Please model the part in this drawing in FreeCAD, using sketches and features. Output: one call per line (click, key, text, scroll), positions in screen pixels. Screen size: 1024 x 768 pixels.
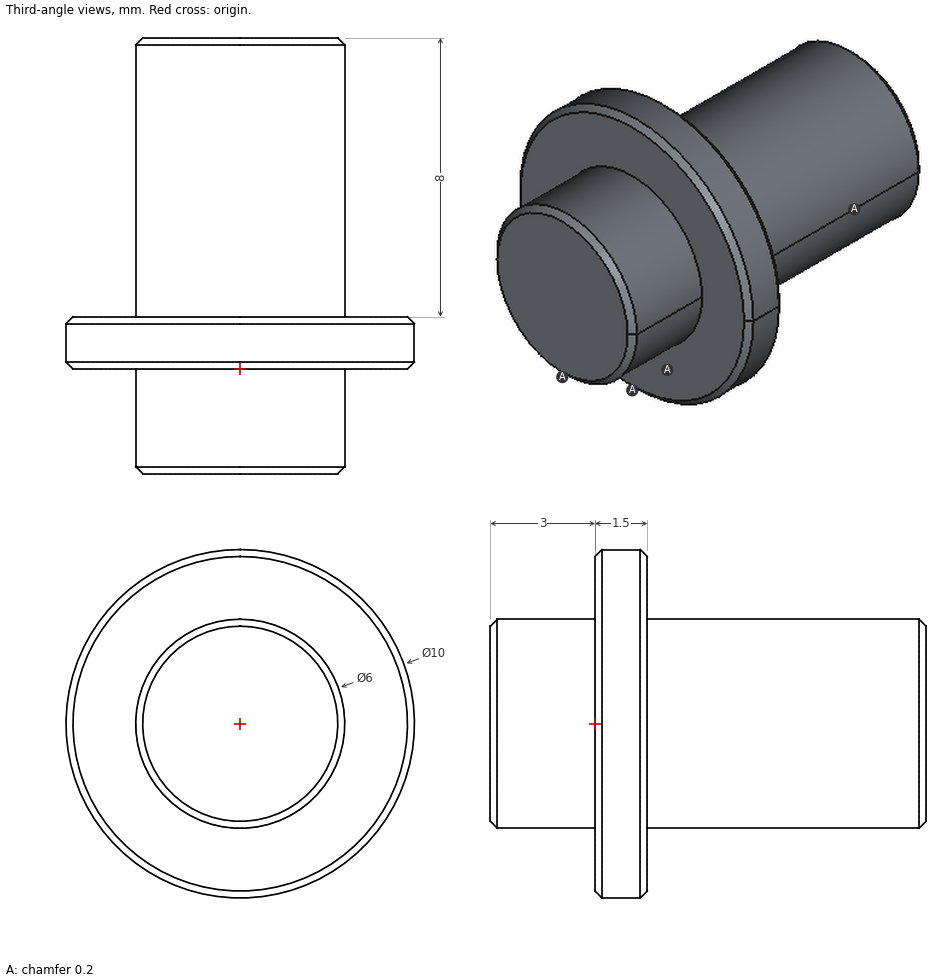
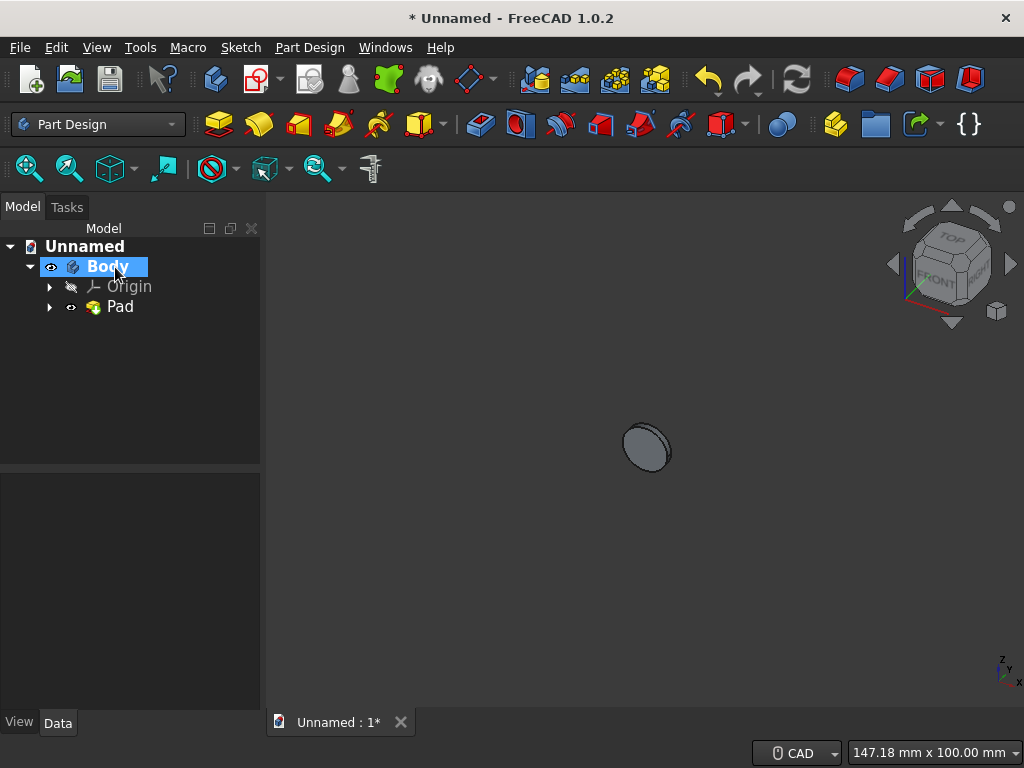
key(v)
key(f)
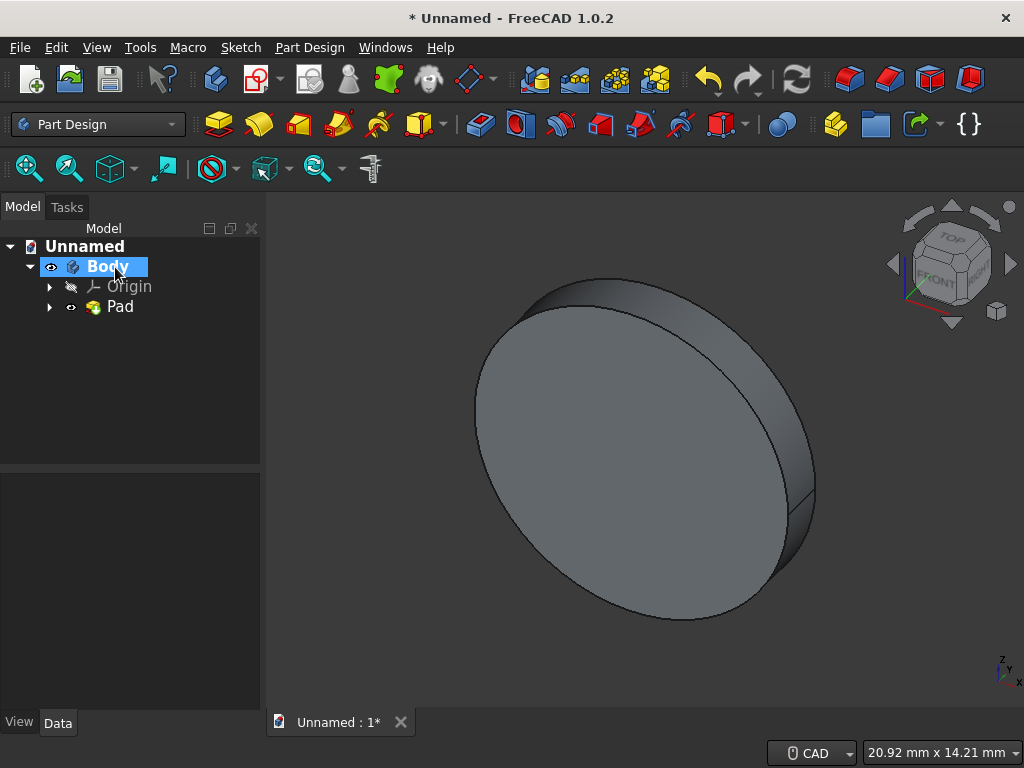
key(4)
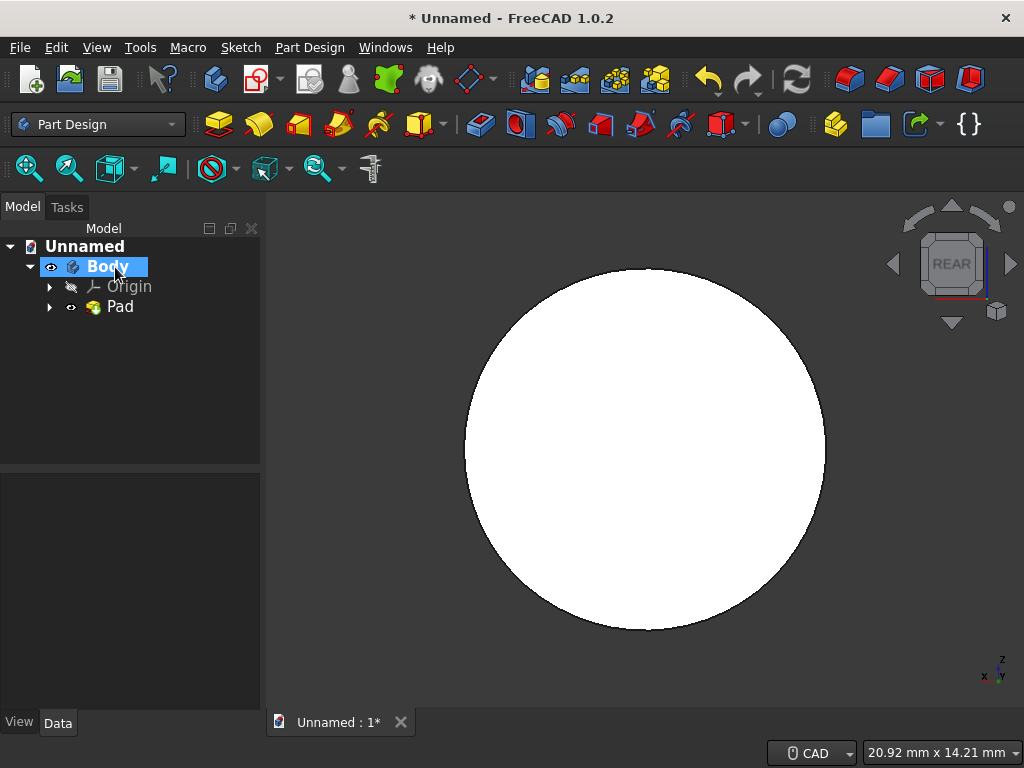
click(645, 449)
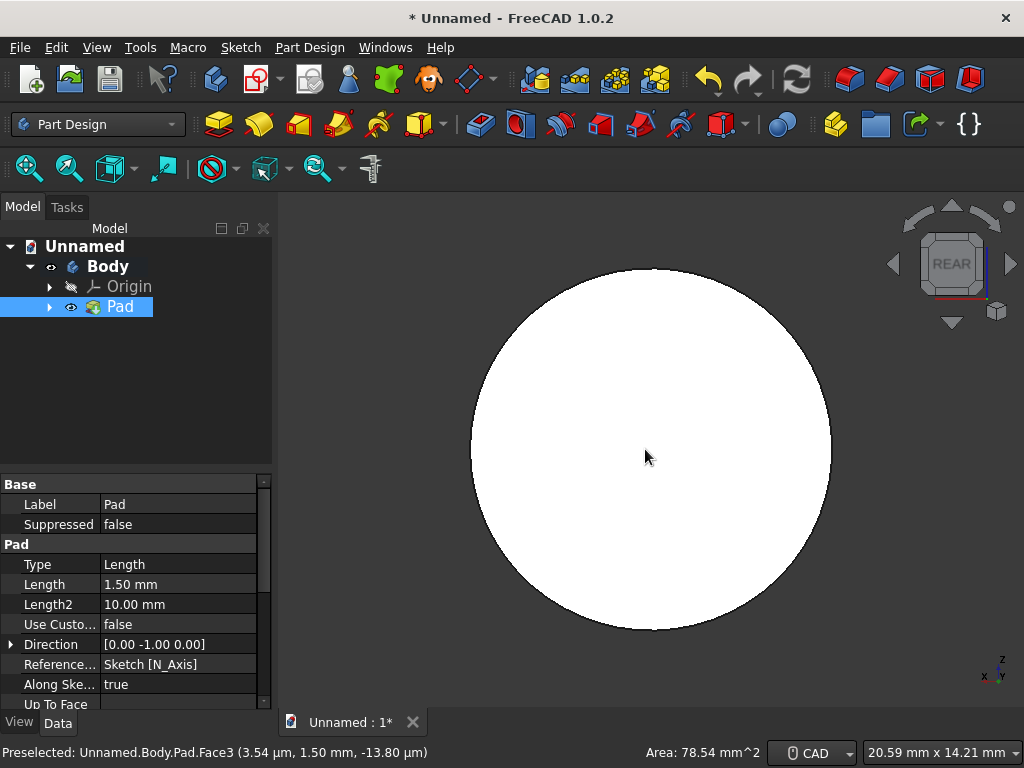
click(256, 80)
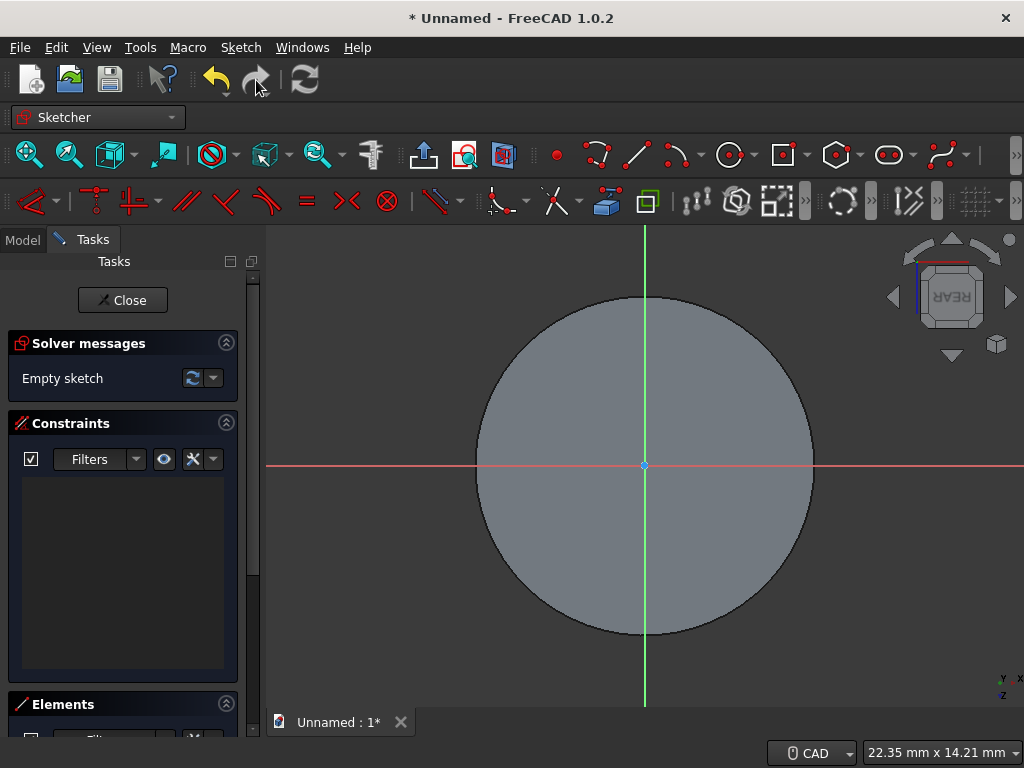
scroll(784, 466, up, 2)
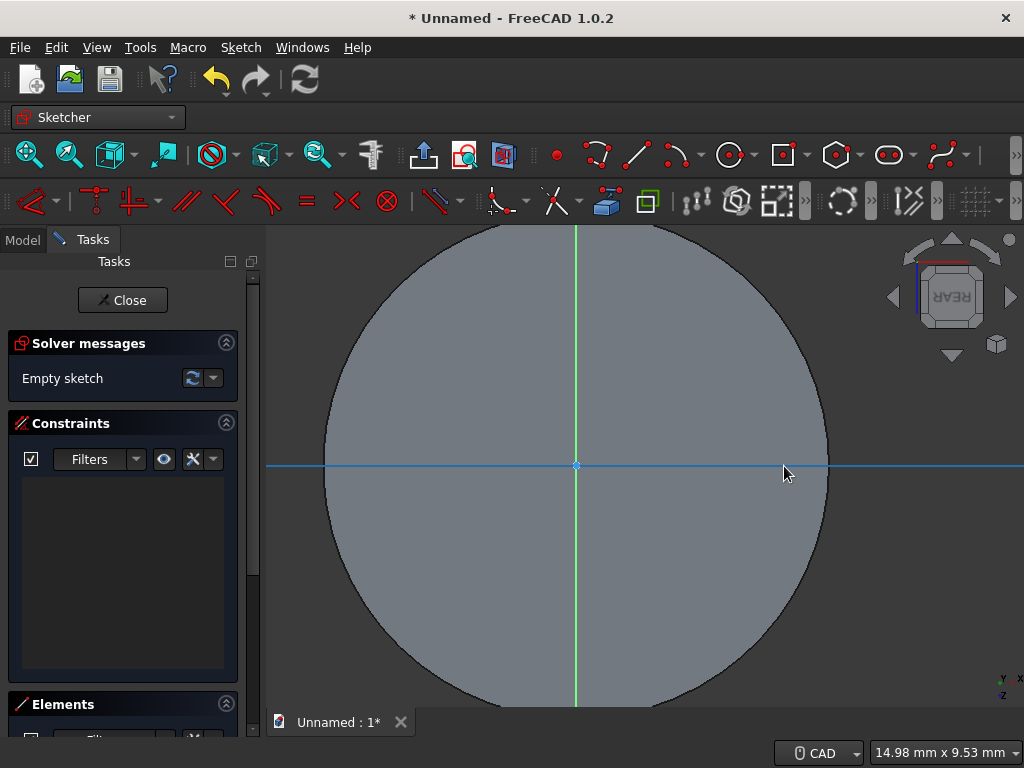
click(730, 156)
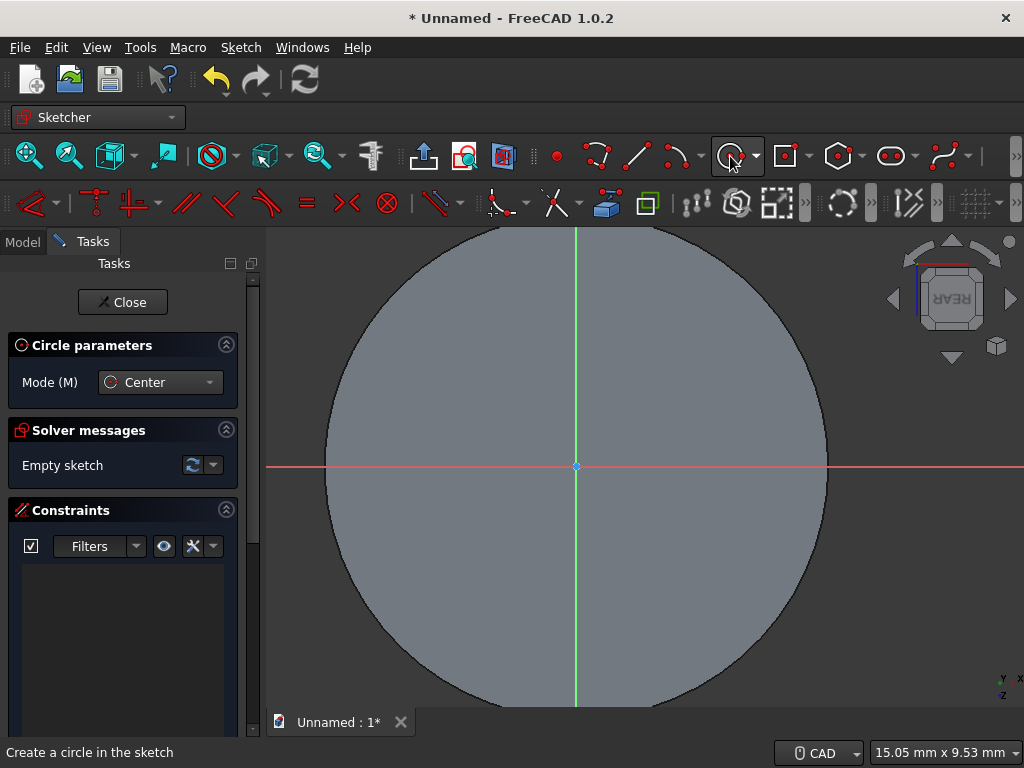
click(576, 467)
move(683, 360)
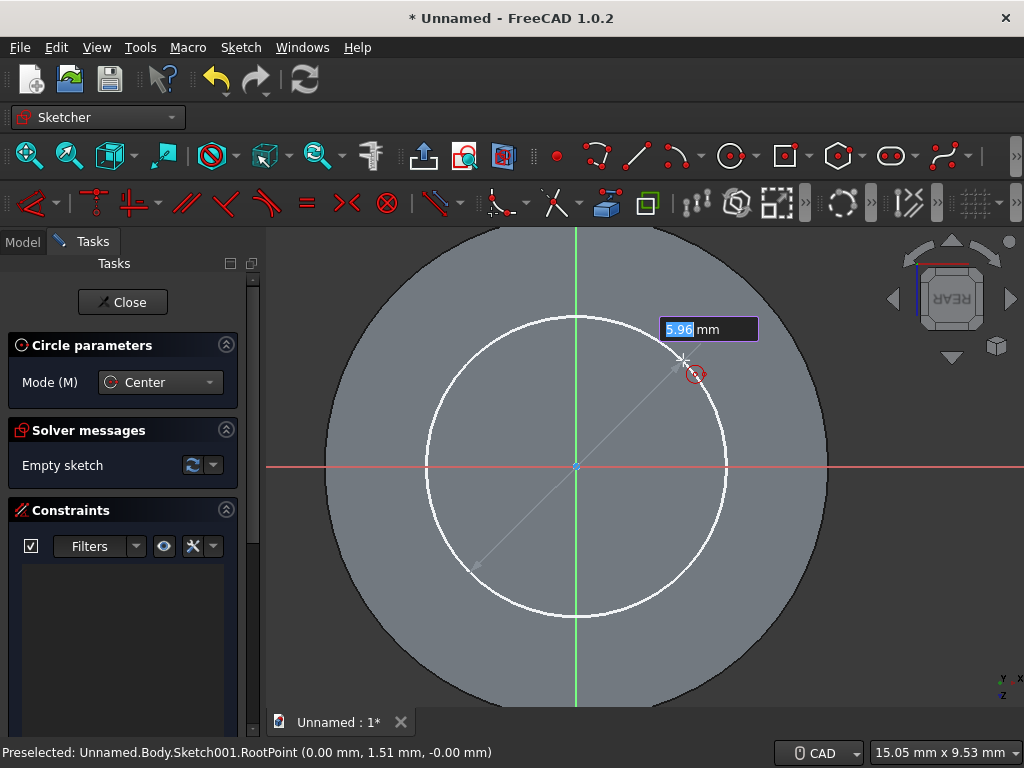
text(6)
key(Return)
key(Escape)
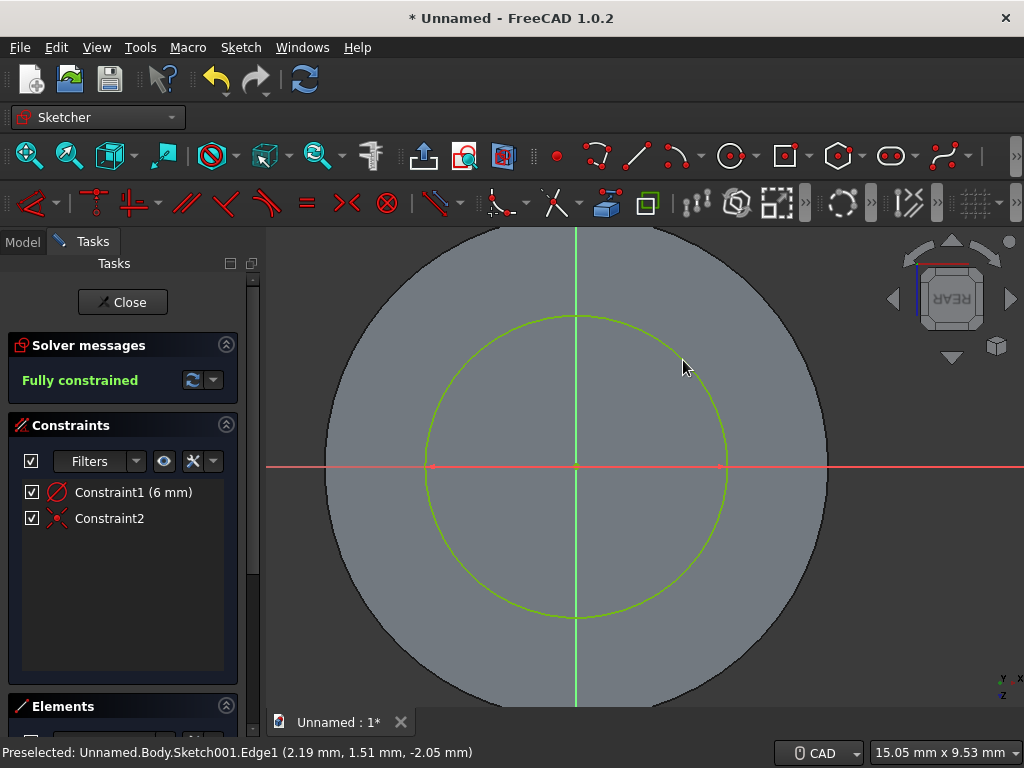
click(123, 302)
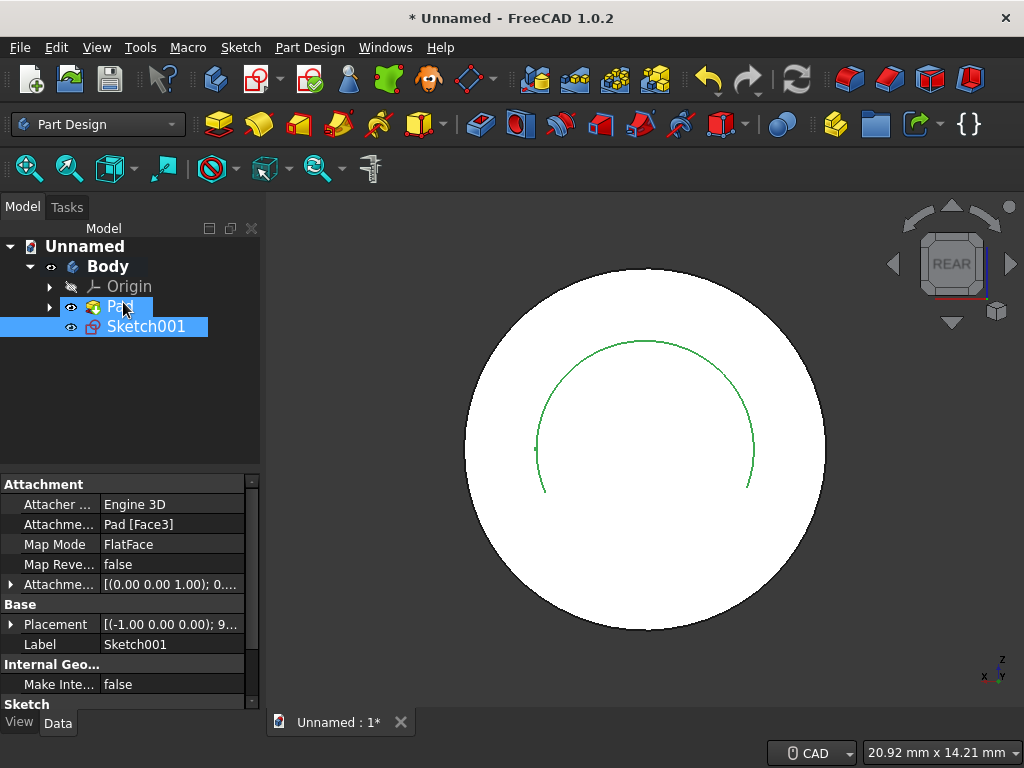
click(220, 124)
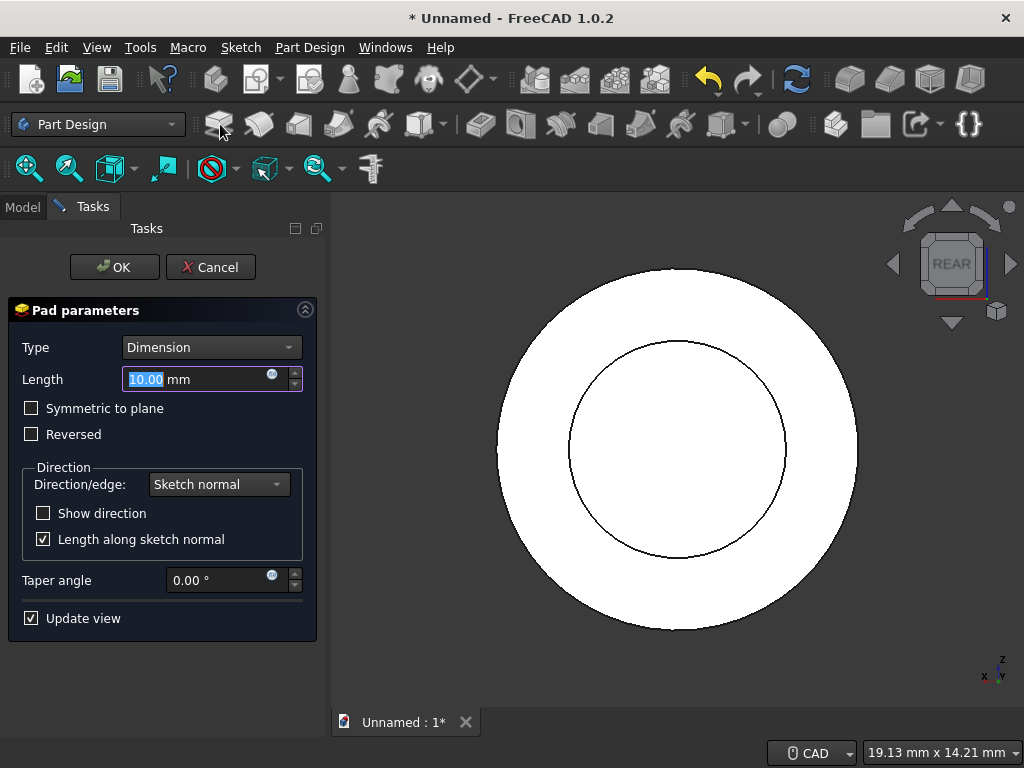
text(8)
key(Tab)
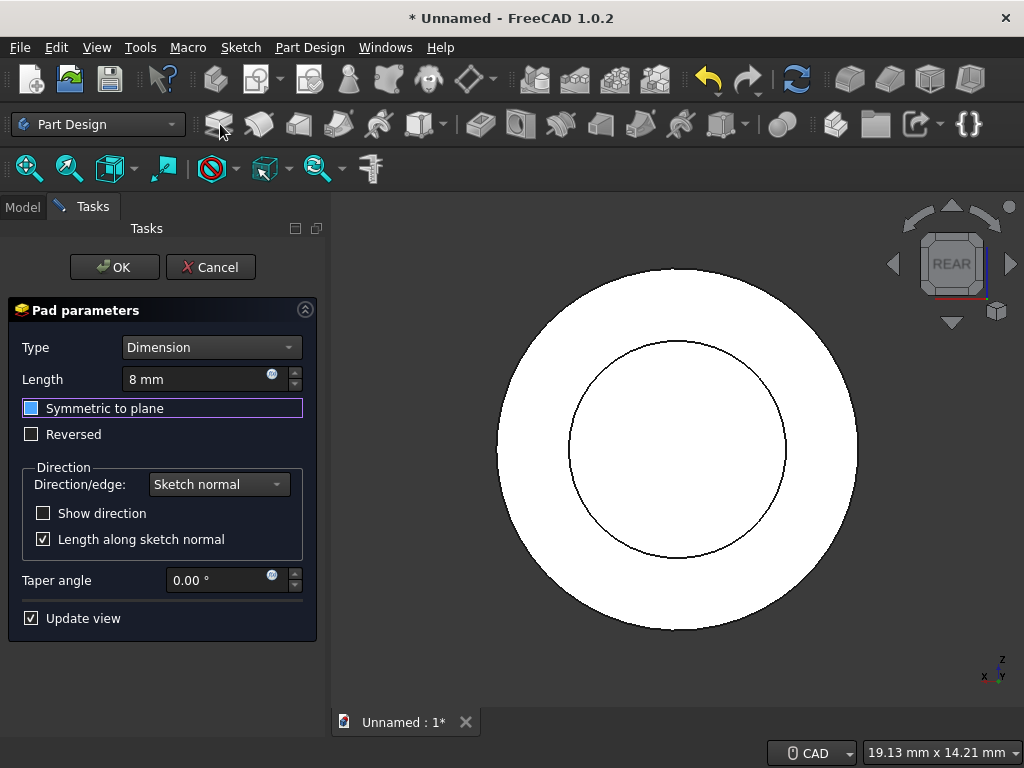
click(115, 267)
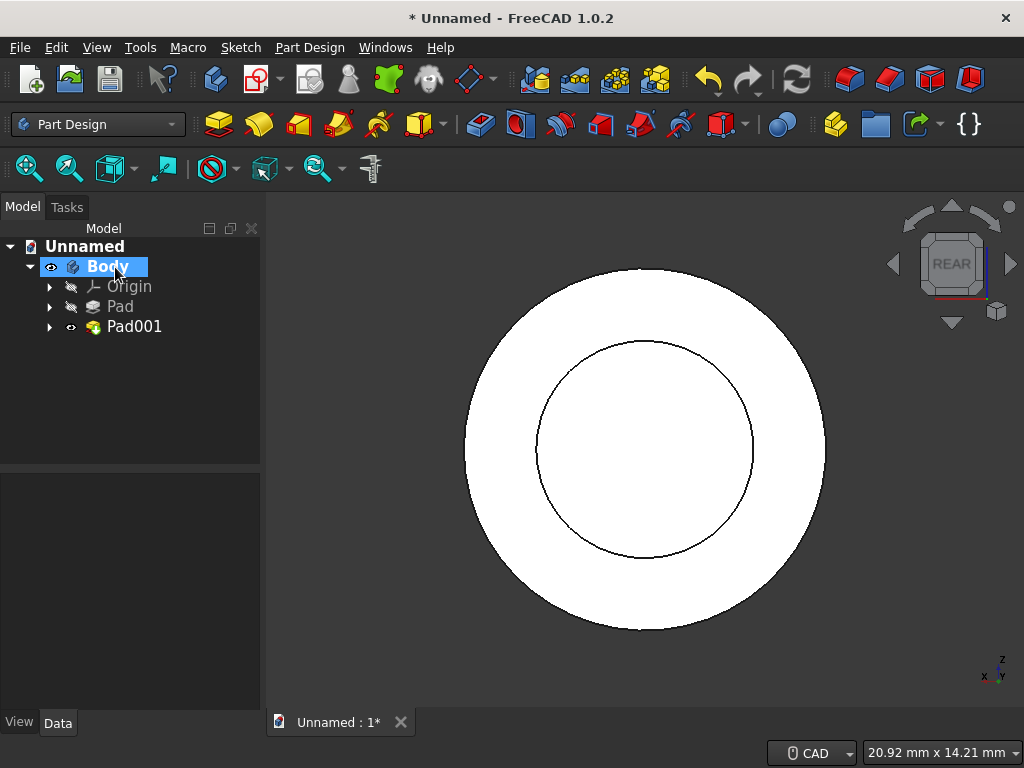
click(50, 287)